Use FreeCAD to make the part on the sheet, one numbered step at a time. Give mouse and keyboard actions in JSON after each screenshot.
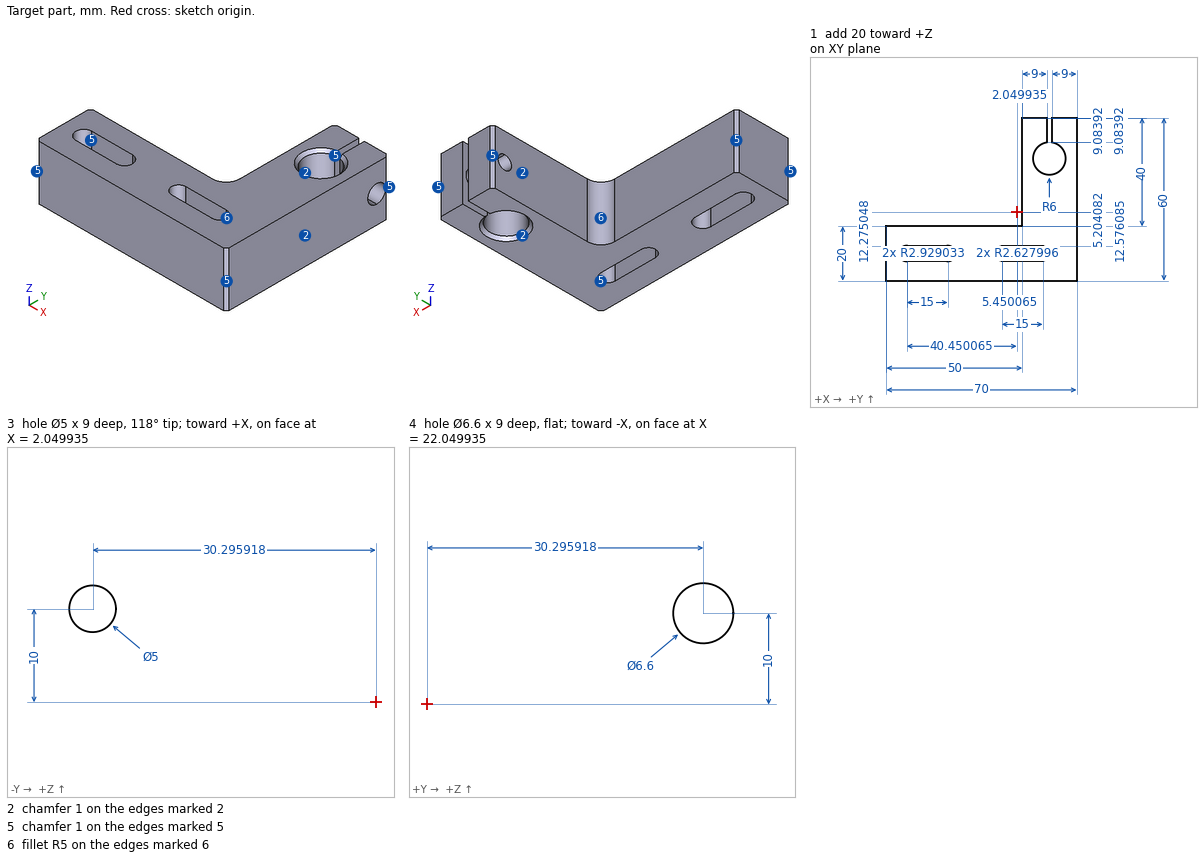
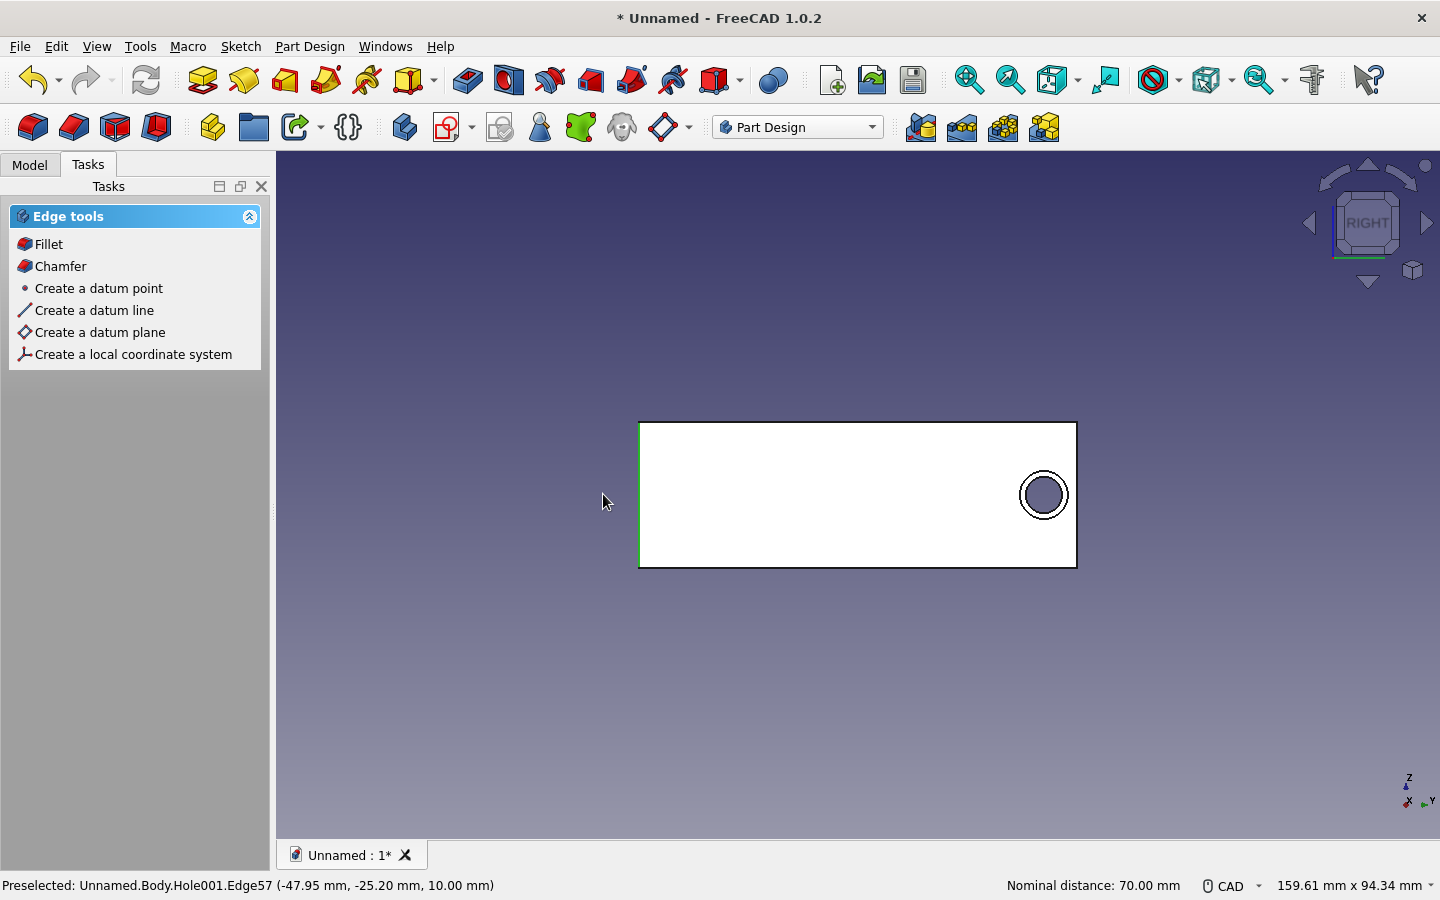
{"action": "left_click", "coordinate": [970, 80]}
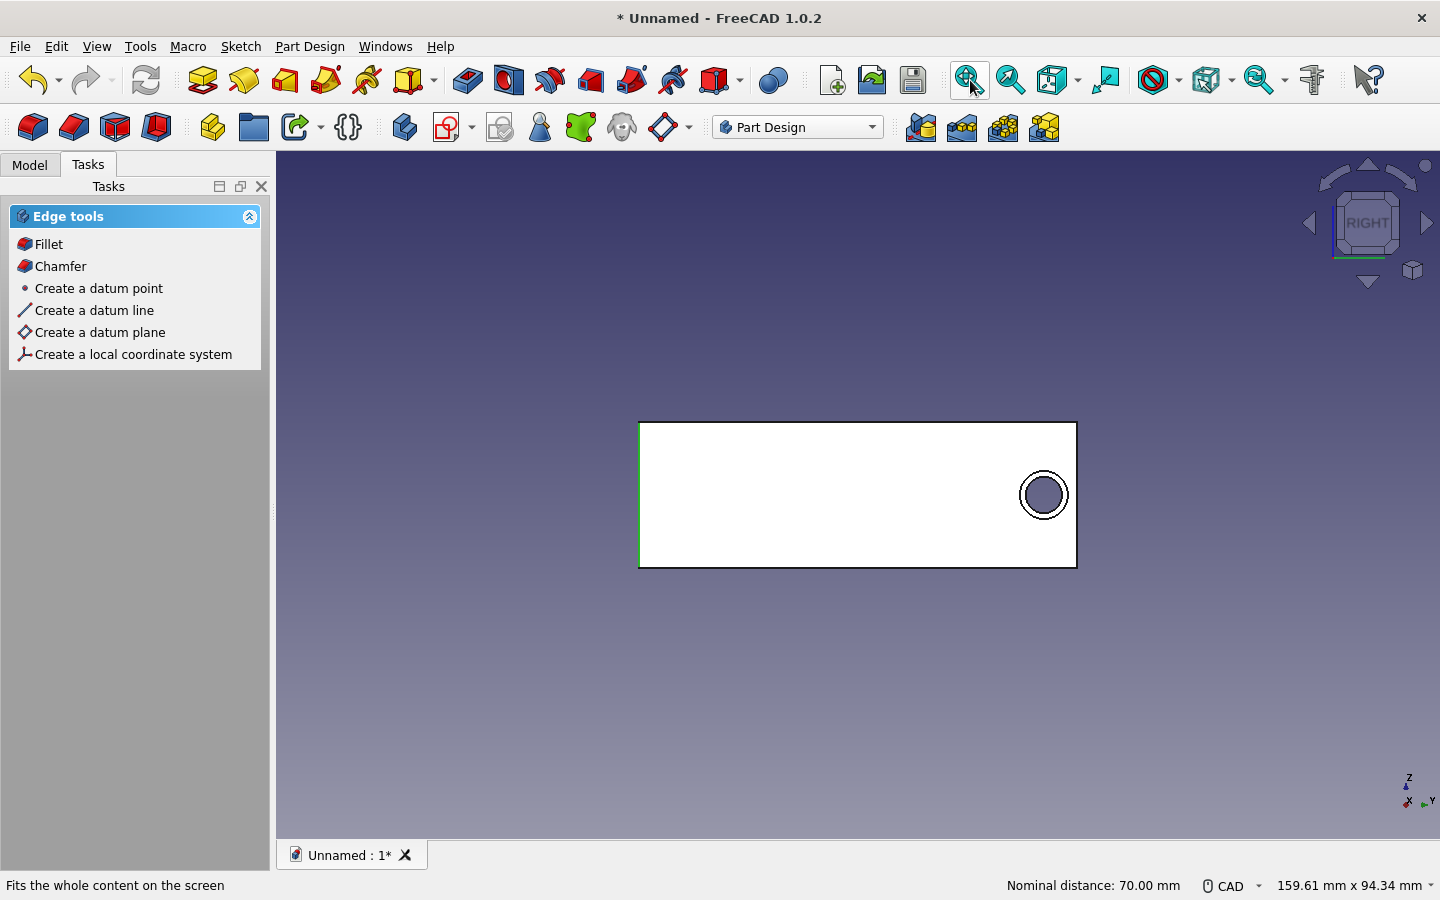
{"action": "left_click", "coordinate": [1077, 494], "text": "ctrl"}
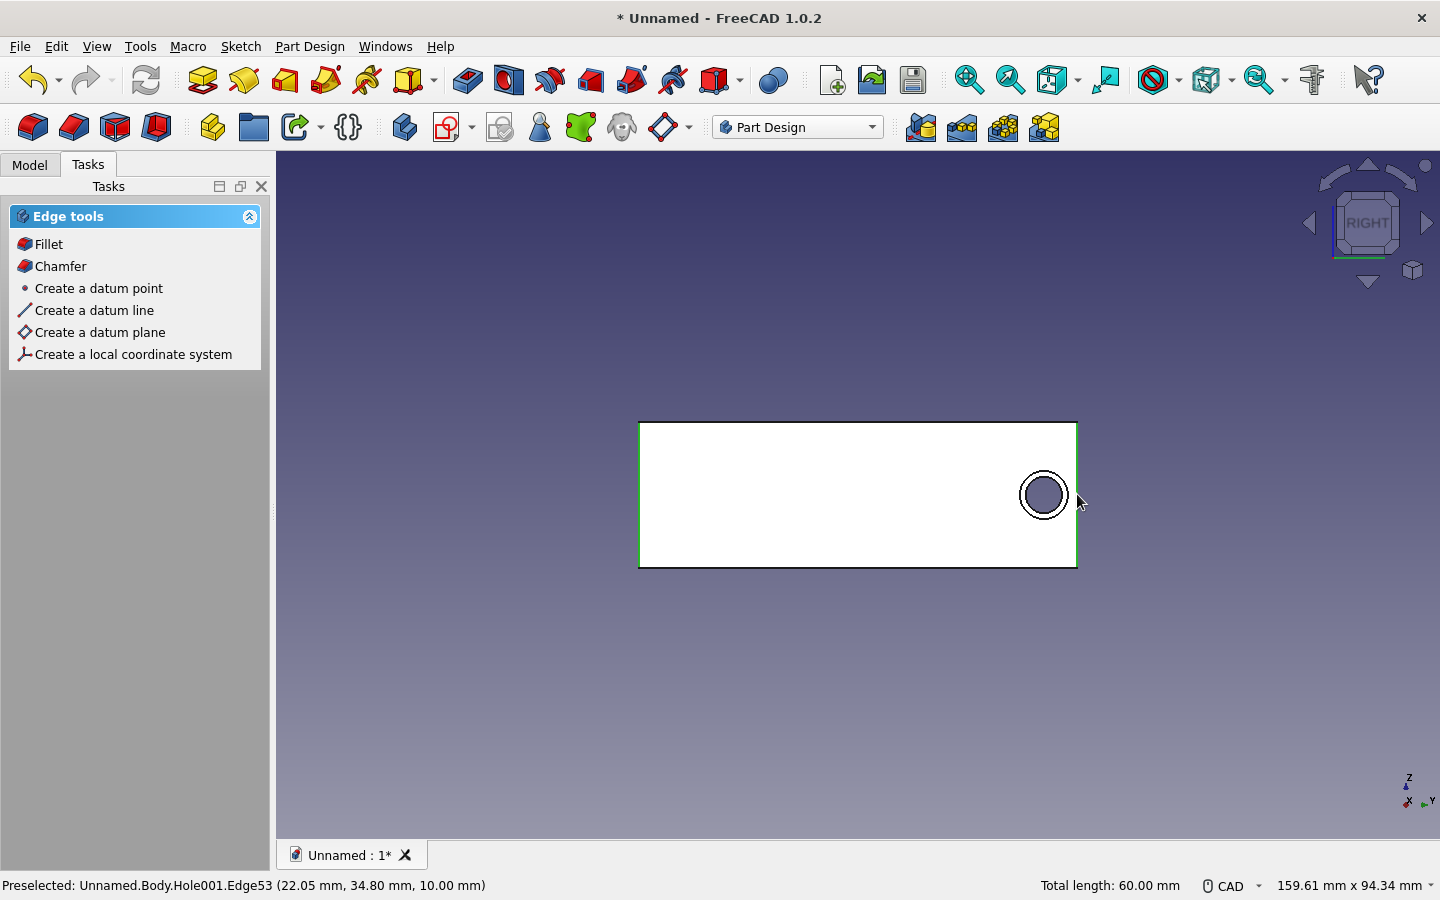
{"action": "key", "text": "5"}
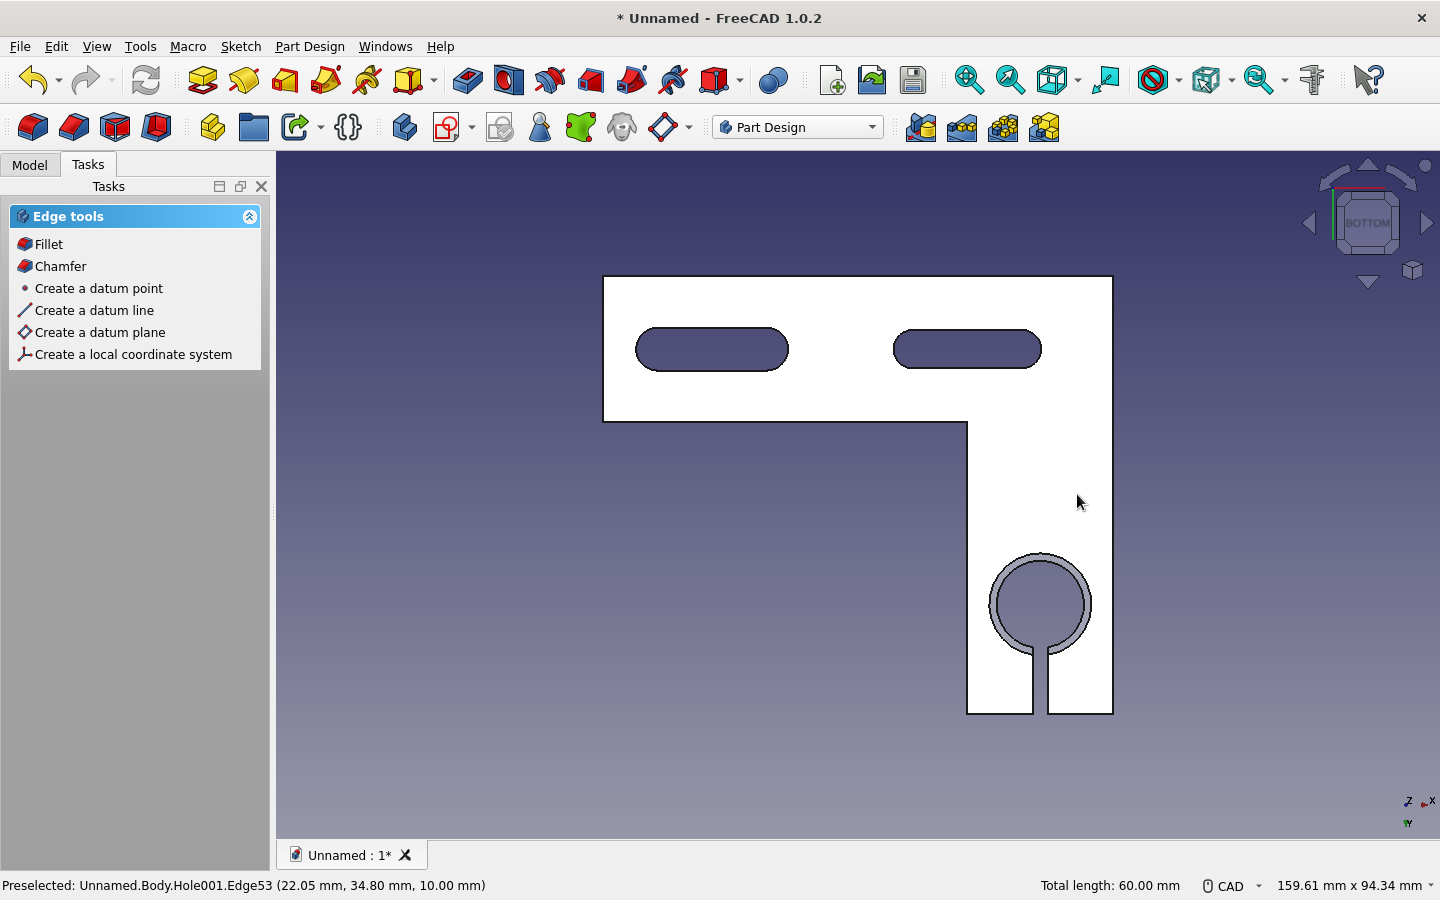
{"action": "key", "text": "4"}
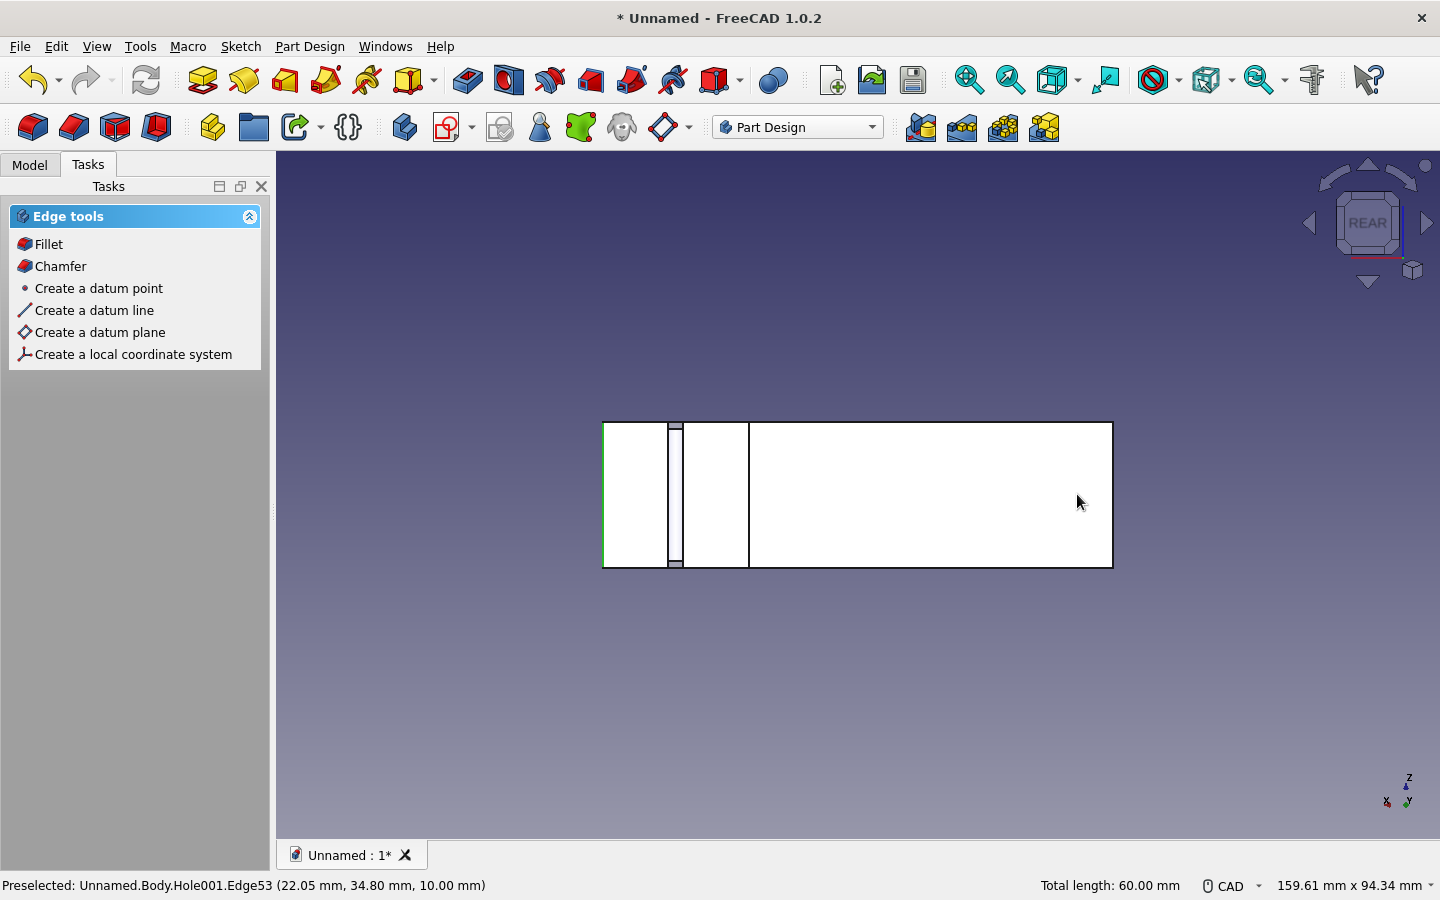
{"action": "left_click", "coordinate": [970, 80]}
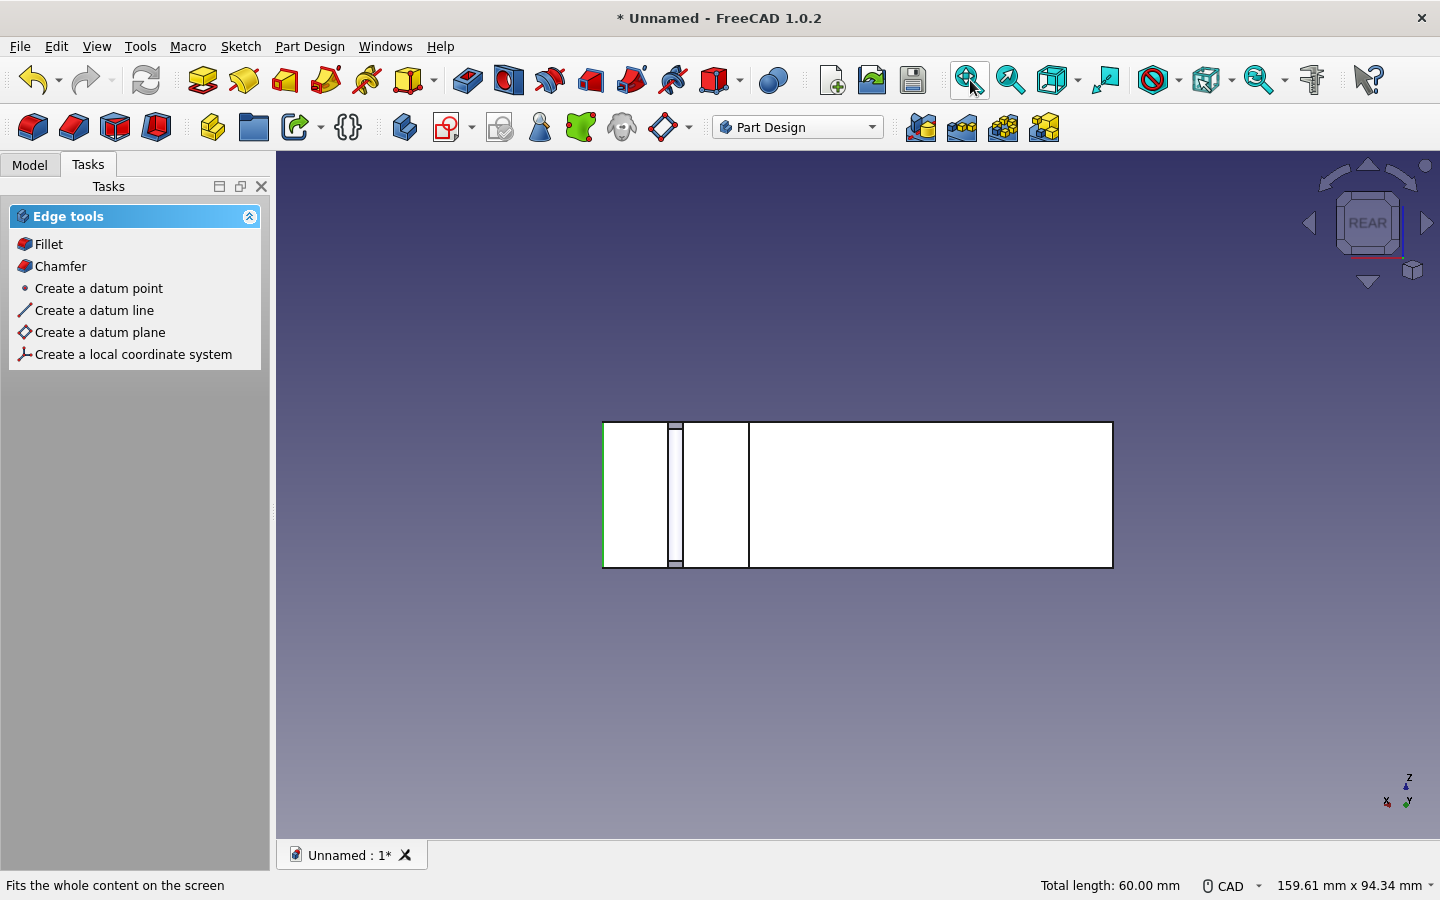
{"action": "left_click", "coordinate": [1113, 494], "text": "ctrl"}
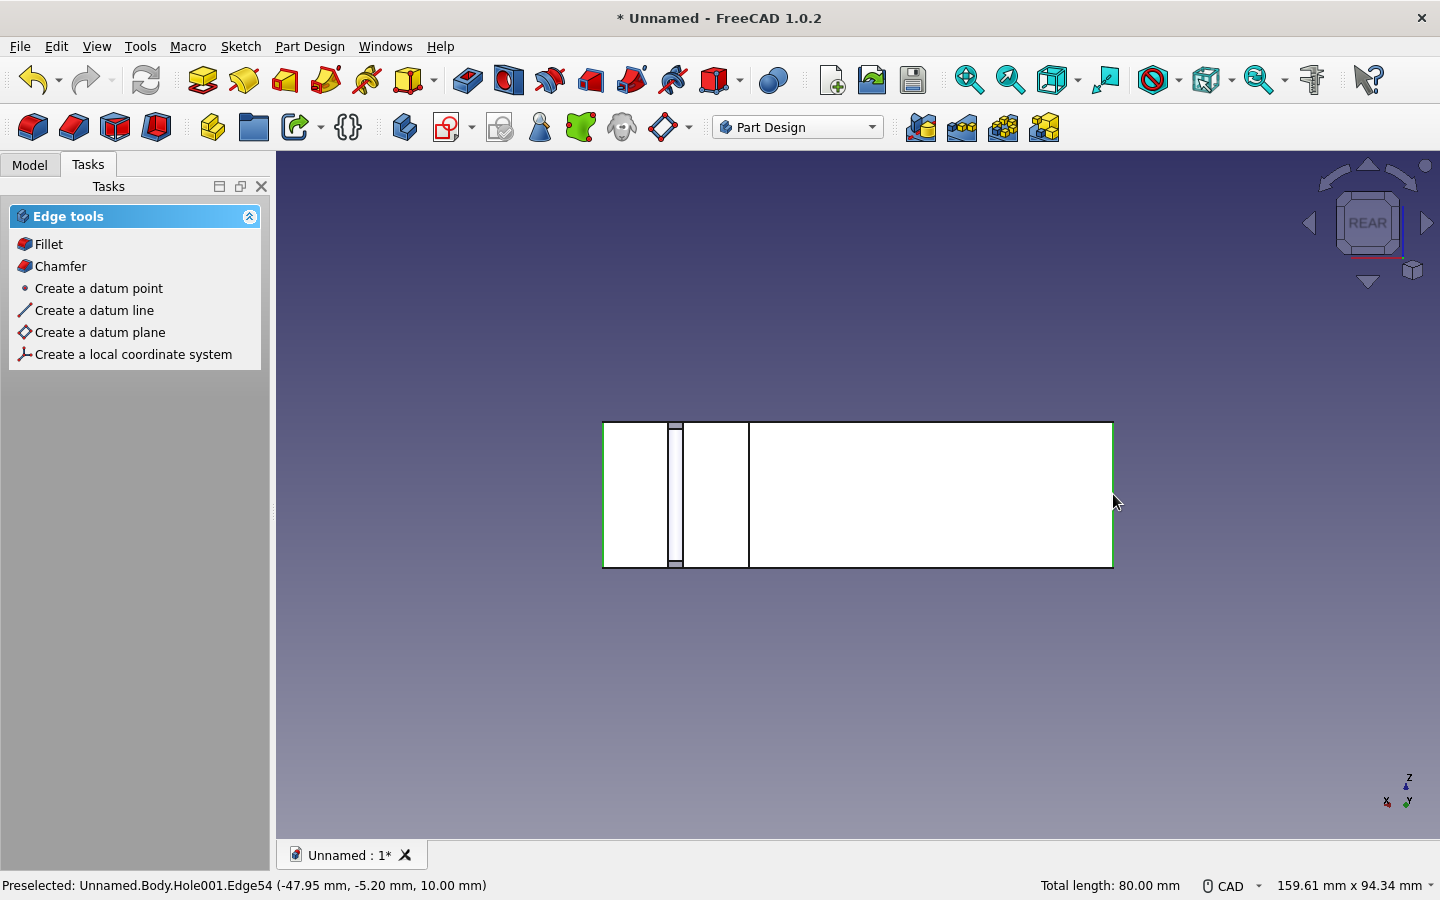
{"action": "left_click", "coordinate": [749, 494], "text": "ctrl"}